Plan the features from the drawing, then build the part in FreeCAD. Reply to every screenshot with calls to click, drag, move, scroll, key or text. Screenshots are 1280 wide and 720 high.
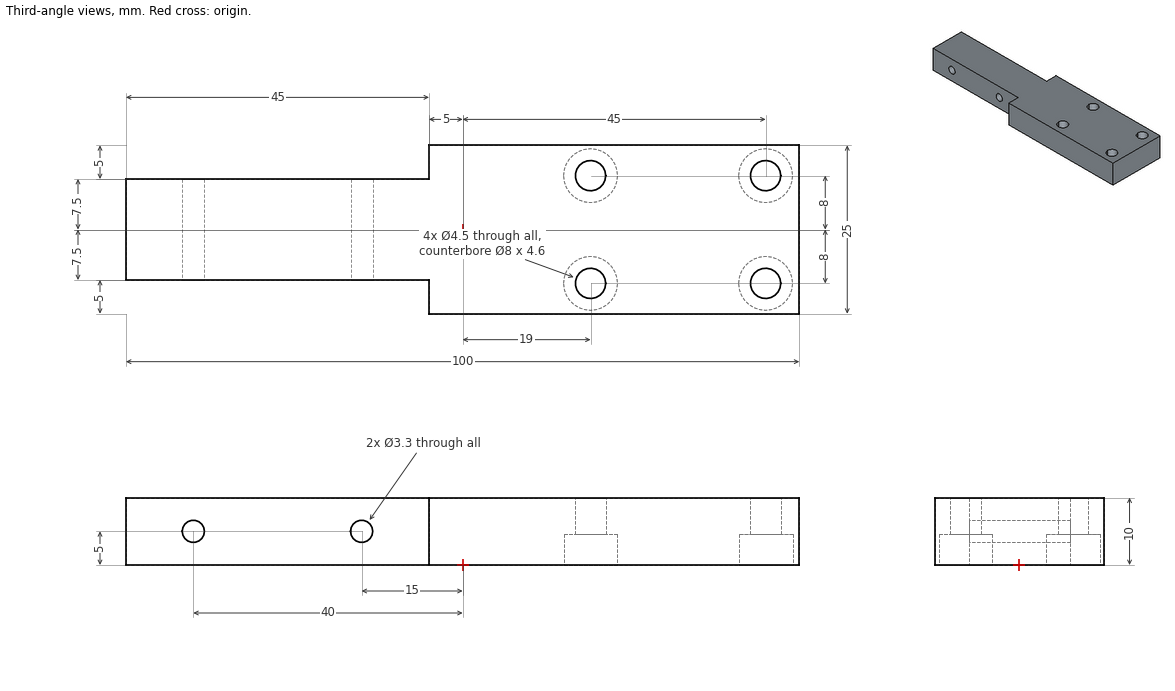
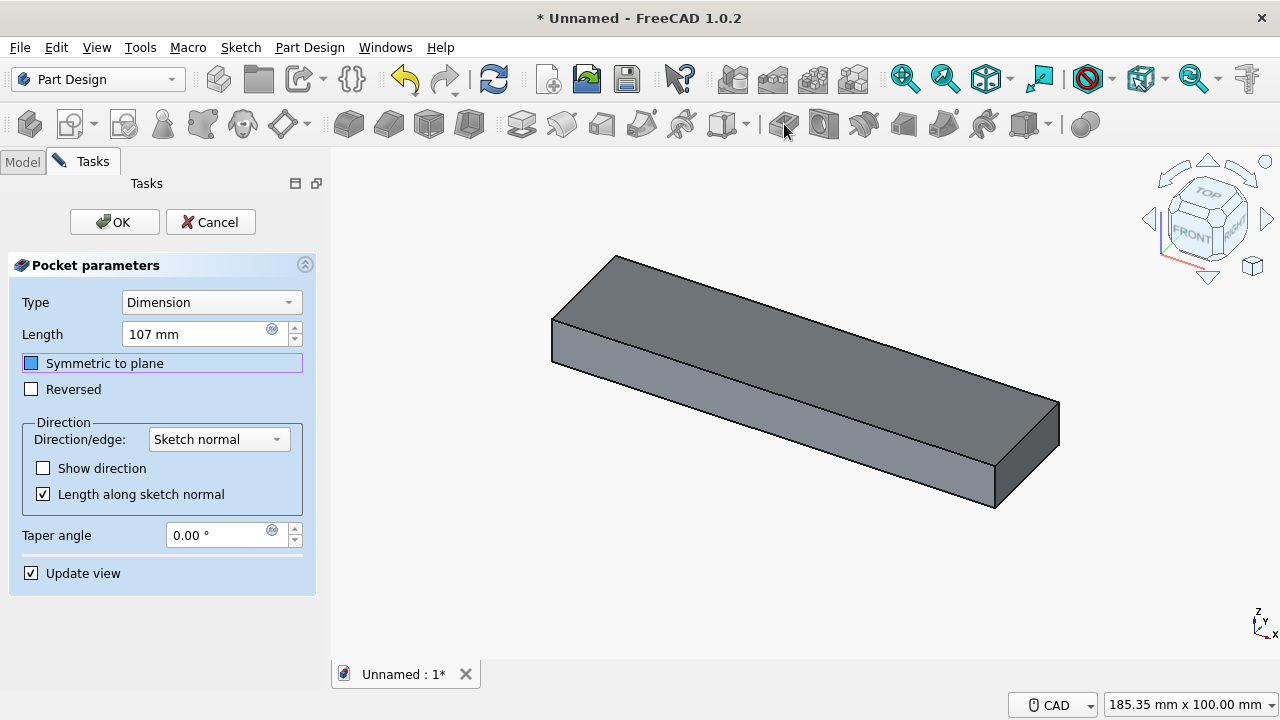
click(30, 363)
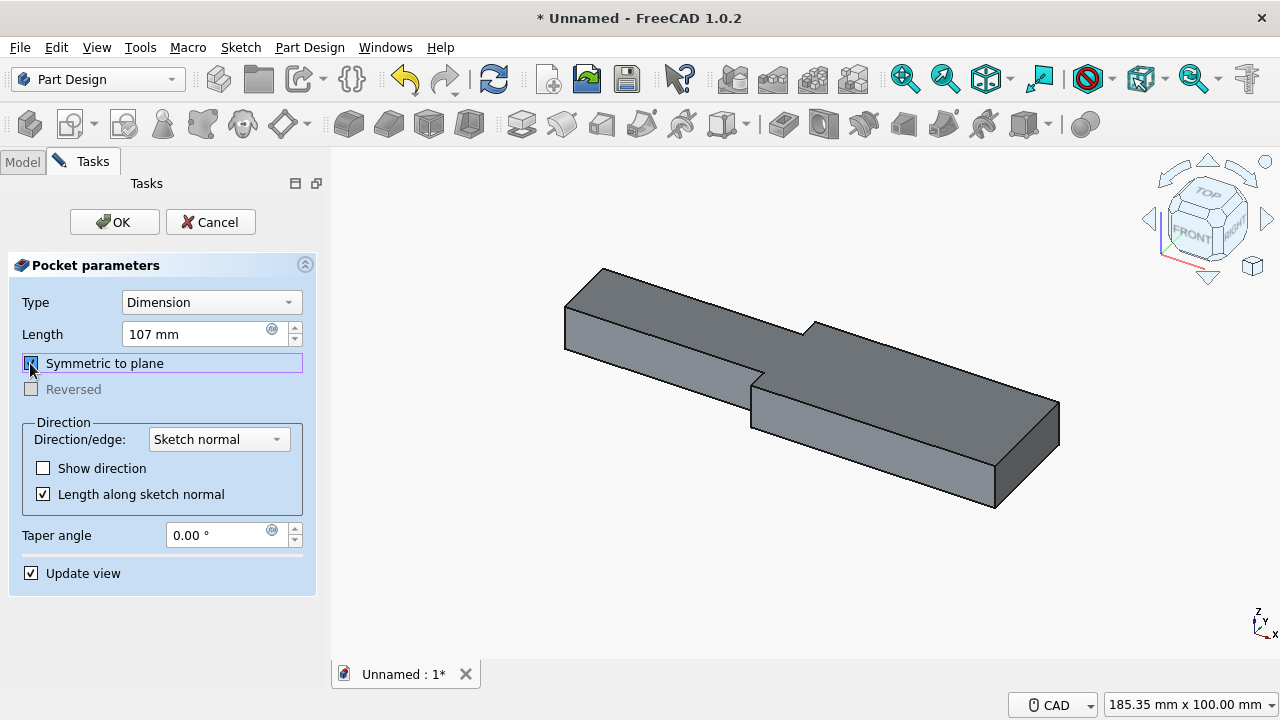
click(115, 222)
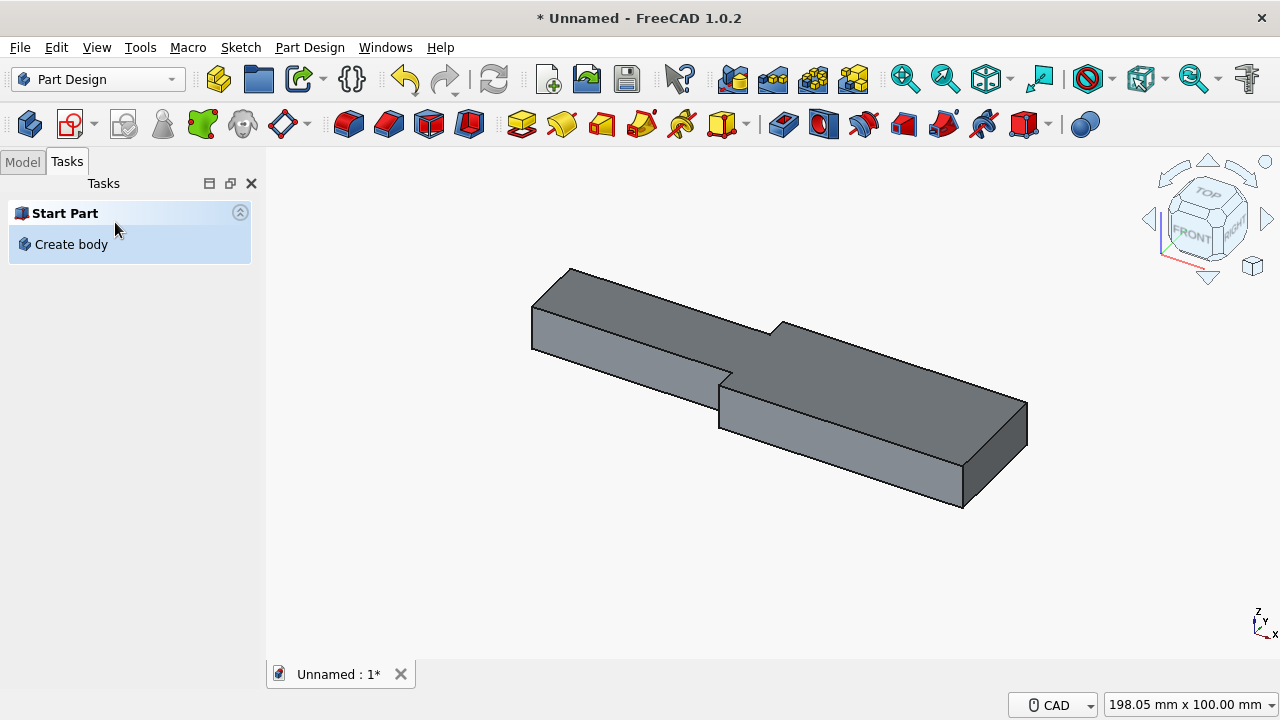
key(5)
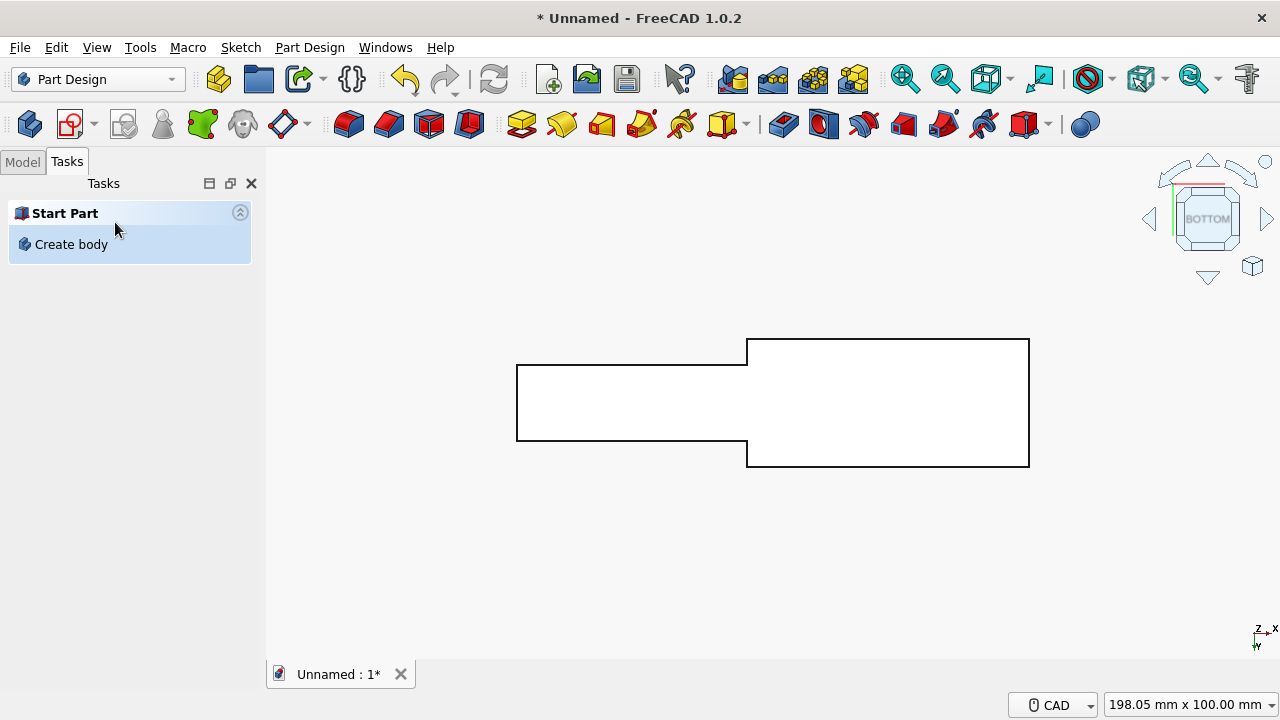
click(919, 402)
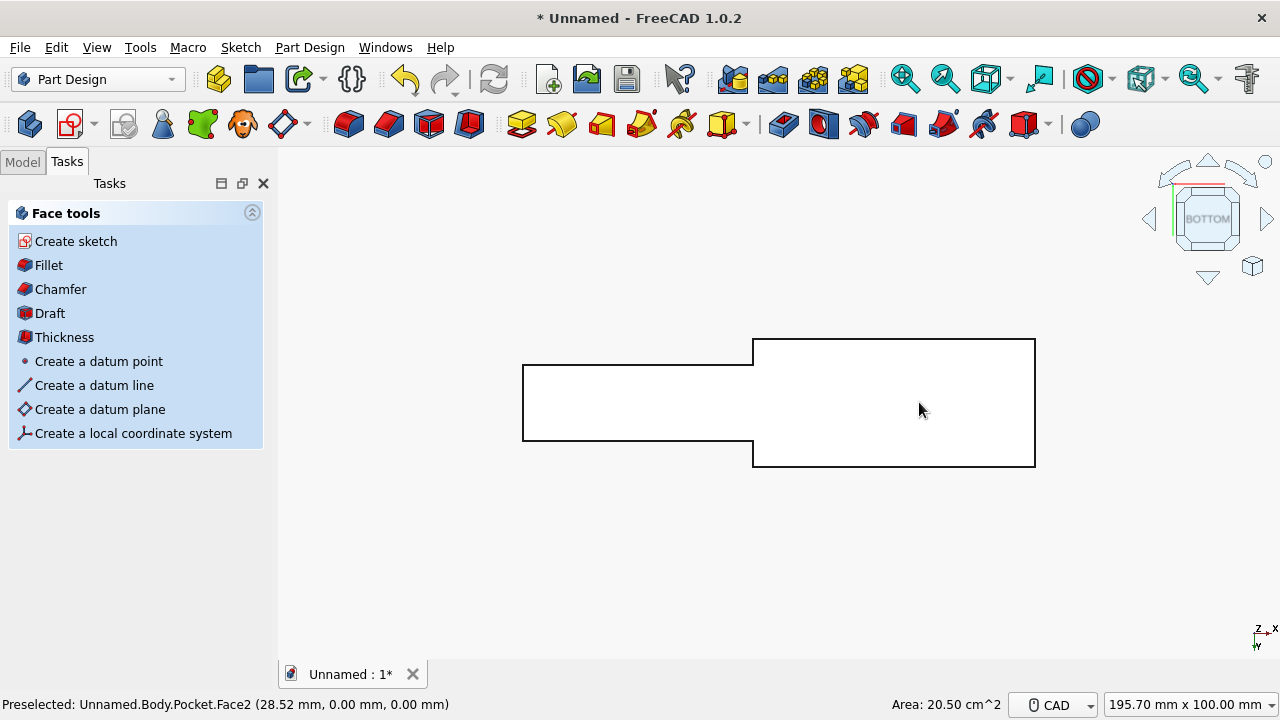
click(70, 124)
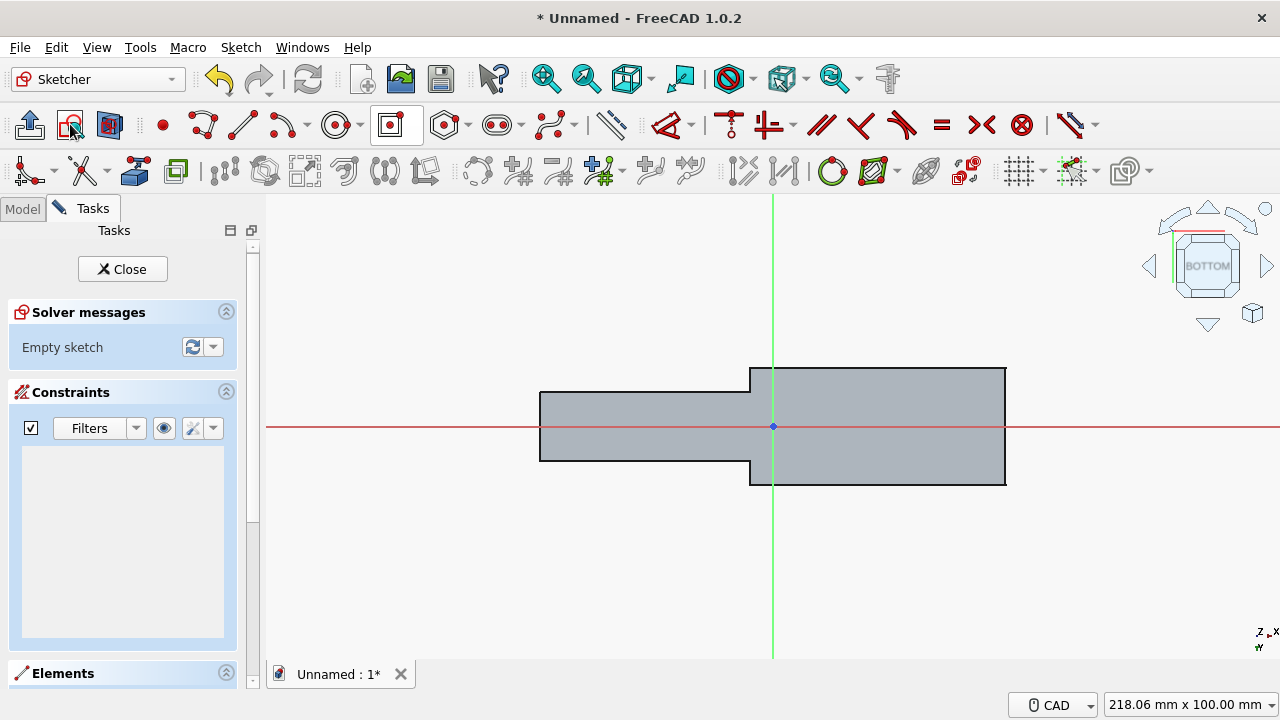
scroll(987, 426, up, 5)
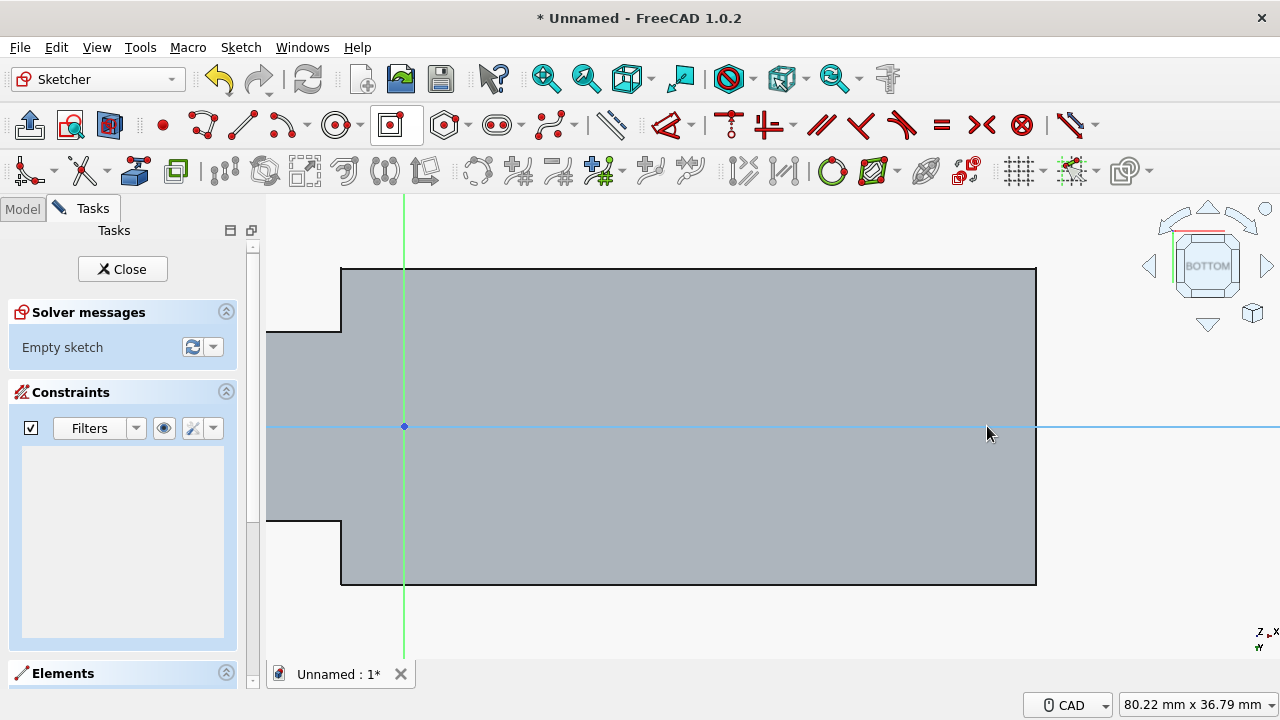
click(336, 126)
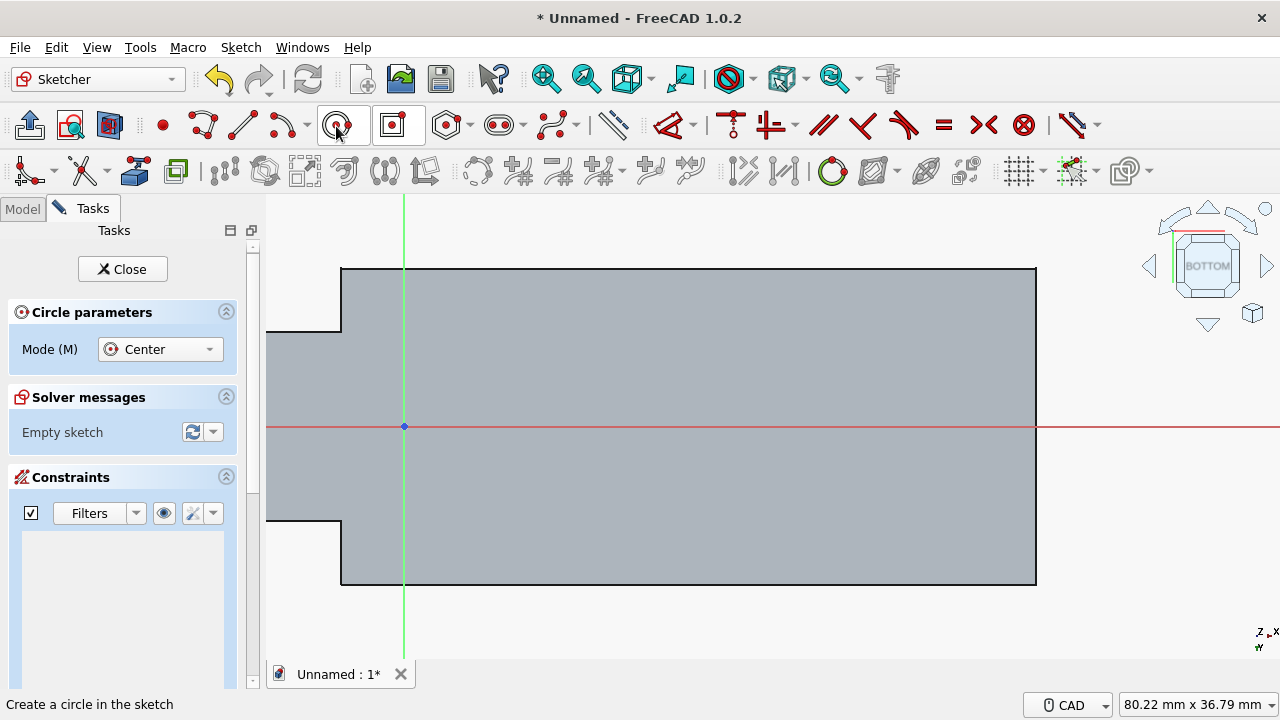
click(644, 325)
click(664, 305)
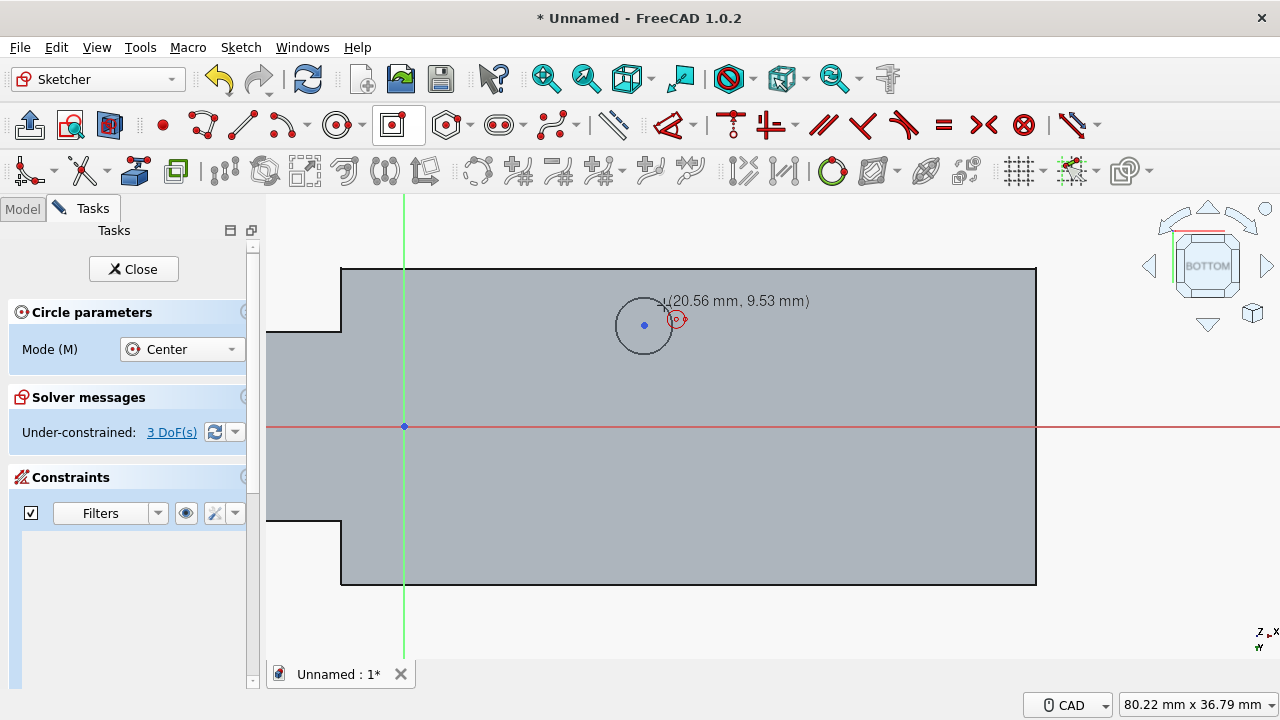
click(644, 528)
click(664, 508)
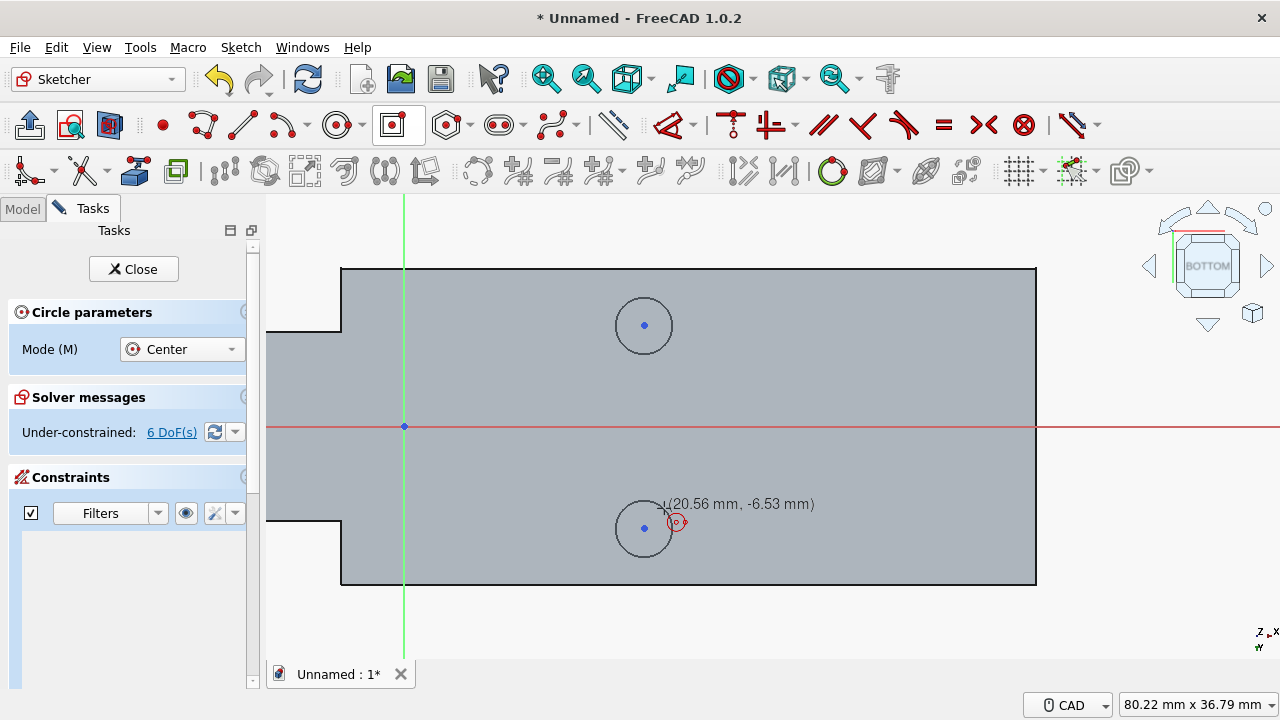
click(973, 528)
click(993, 508)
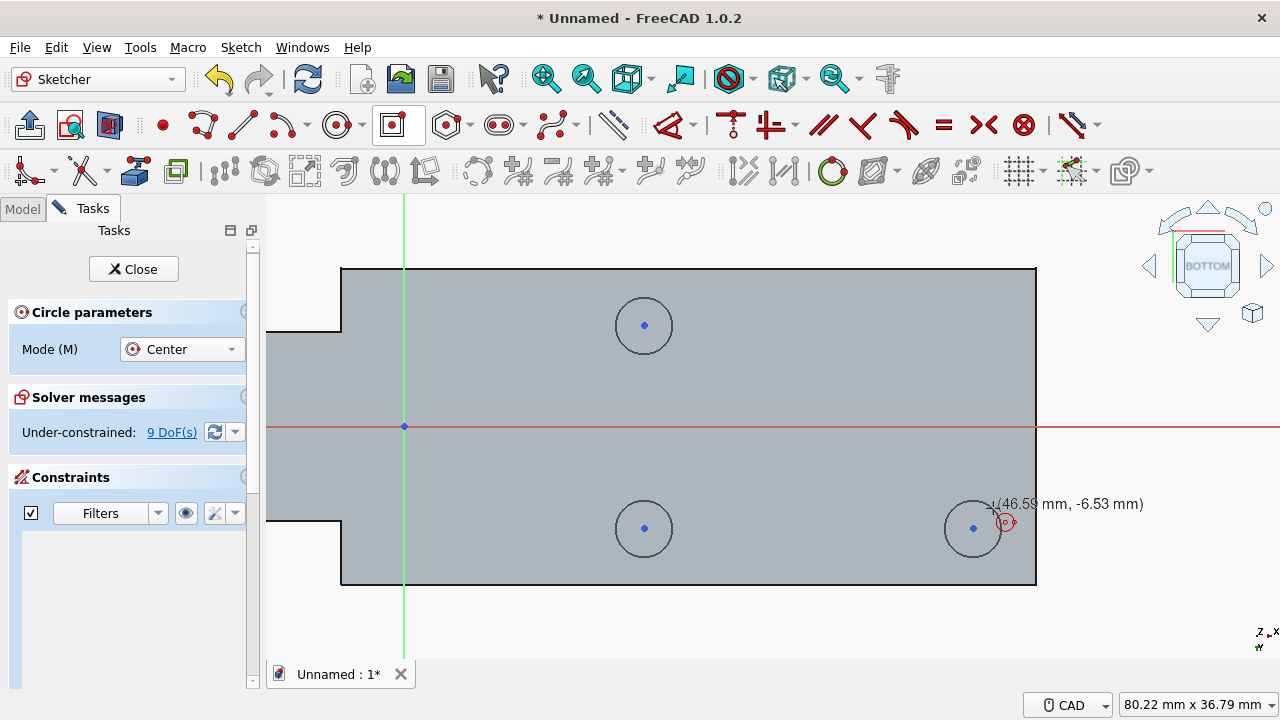
click(973, 325)
click(993, 305)
key(Escape)